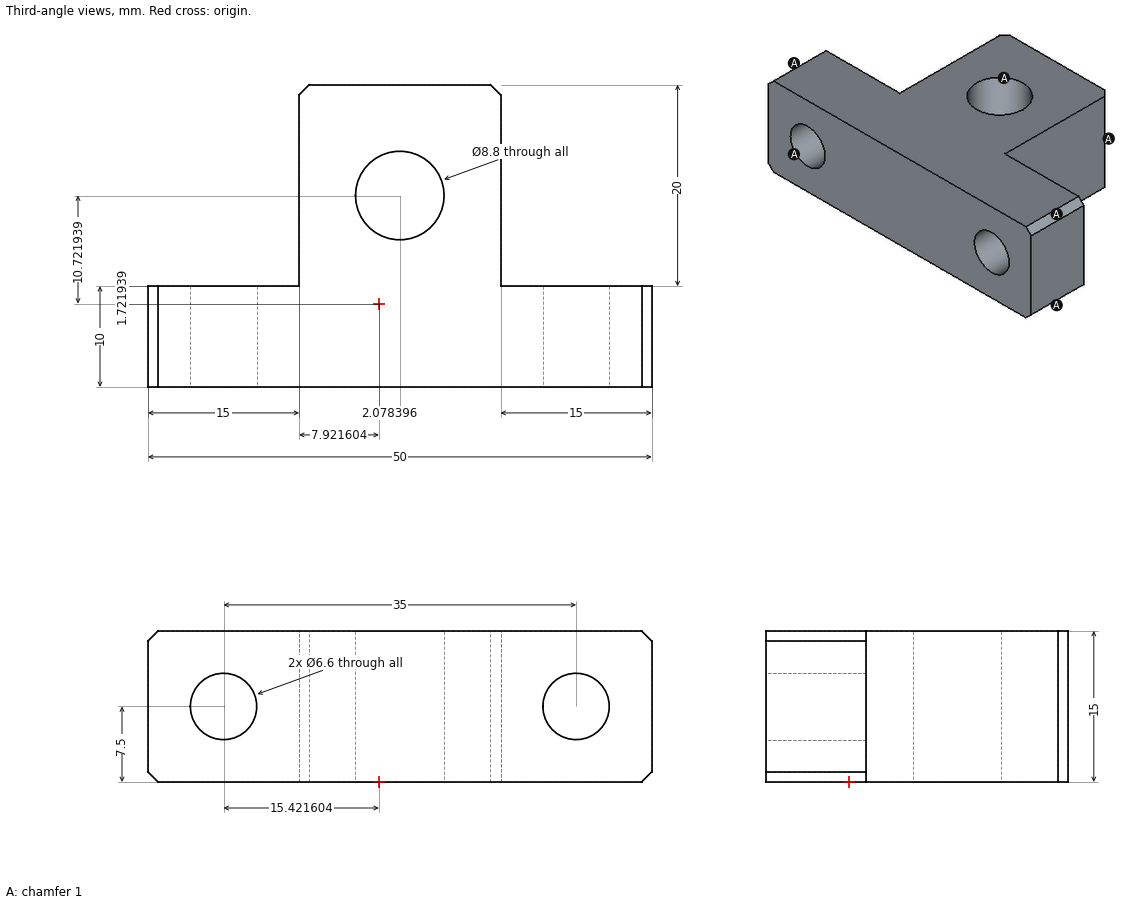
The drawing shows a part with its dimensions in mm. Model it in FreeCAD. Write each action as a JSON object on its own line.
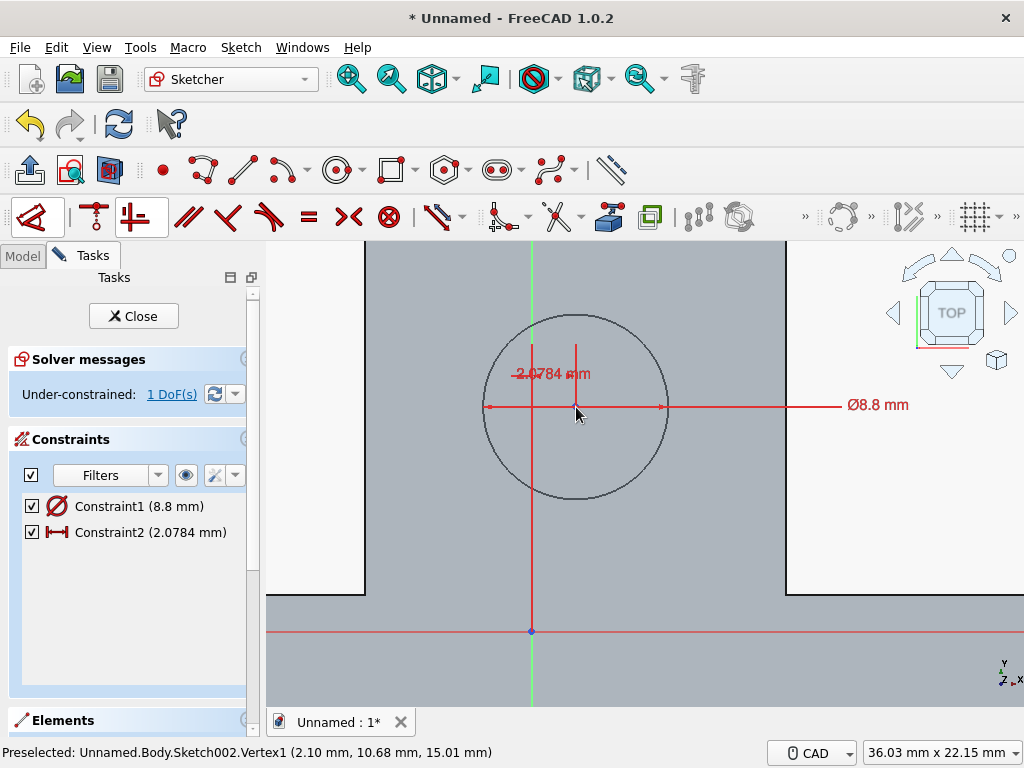
{"action": "left_click", "coordinate": [576, 407]}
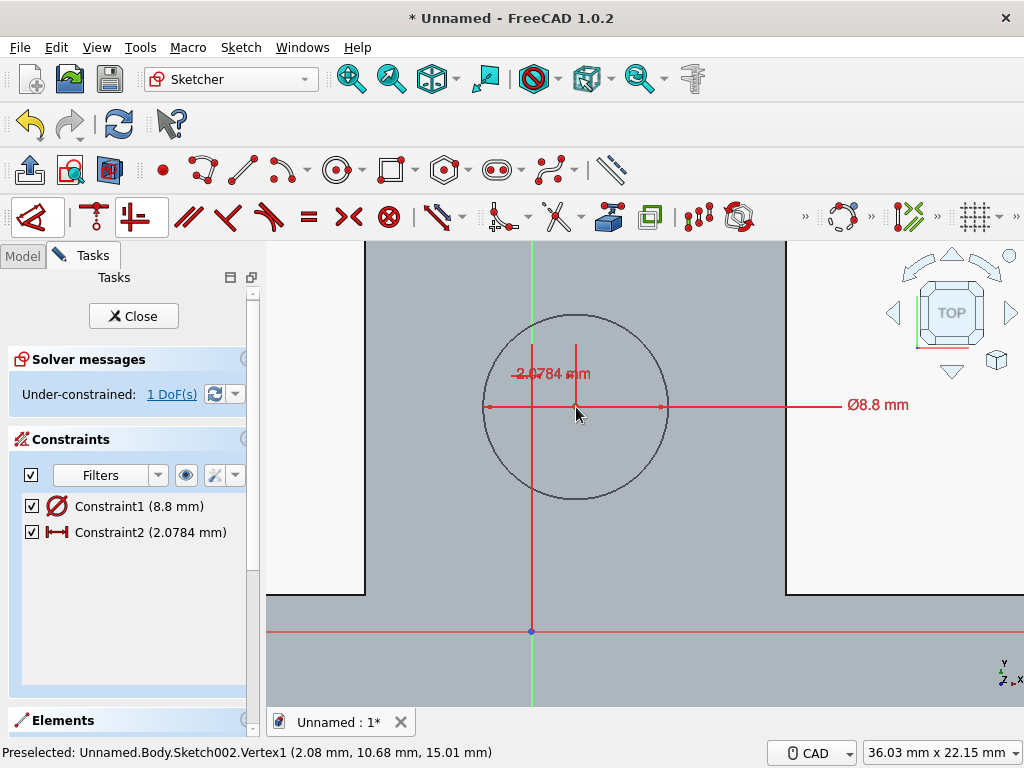
{"action": "left_click", "coordinate": [58, 218]}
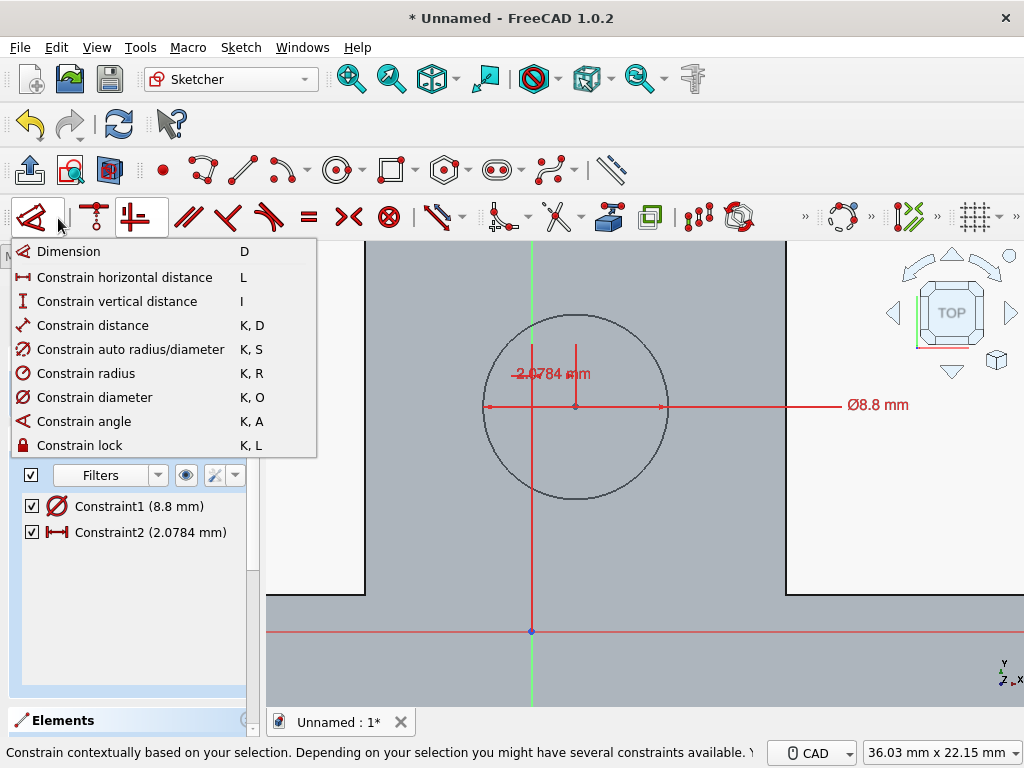
{"action": "left_click", "coordinate": [164, 301]}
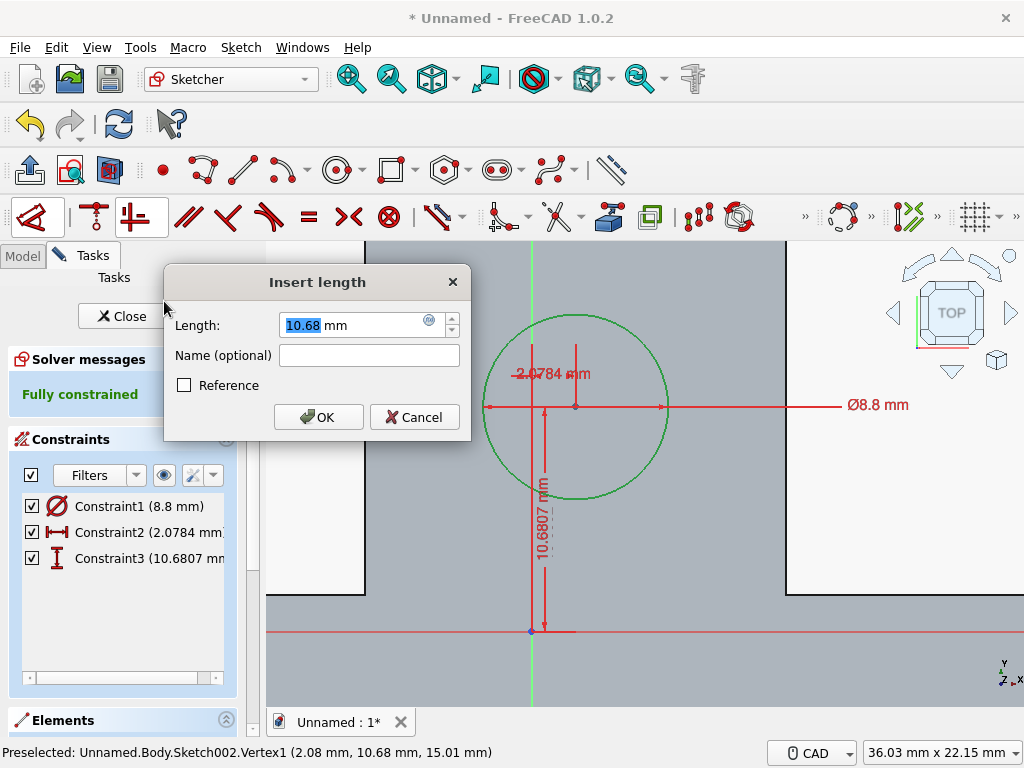
{"action": "type", "text": "10.721939"}
{"action": "key", "text": "Return"}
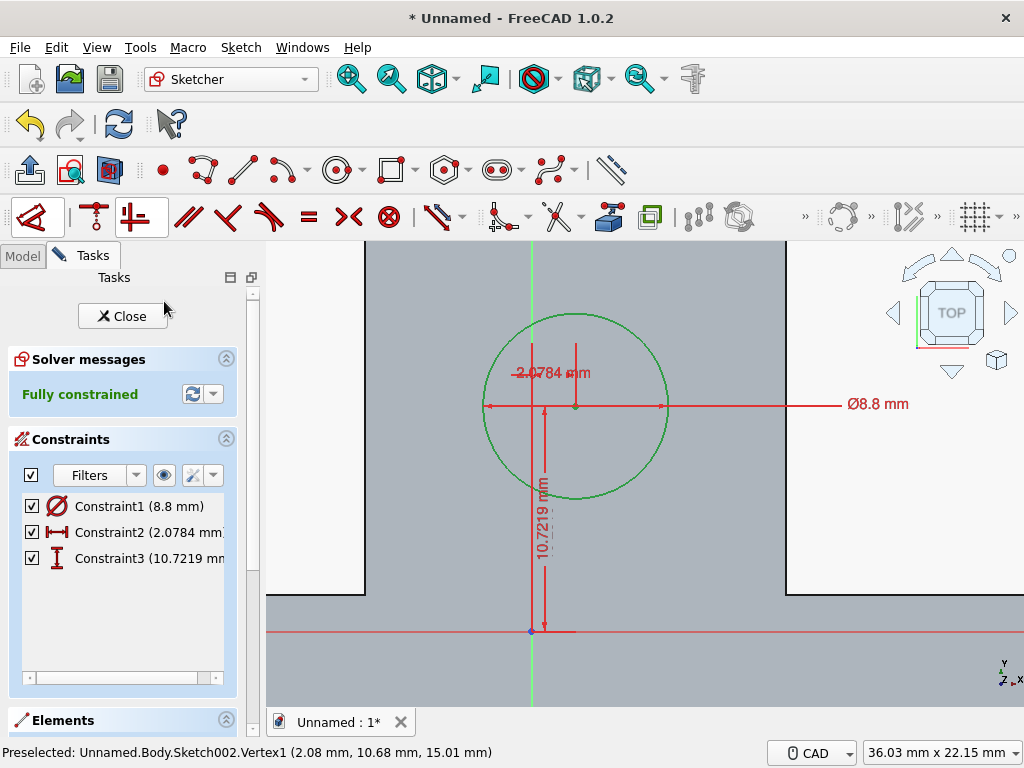
{"action": "left_click", "coordinate": [123, 316]}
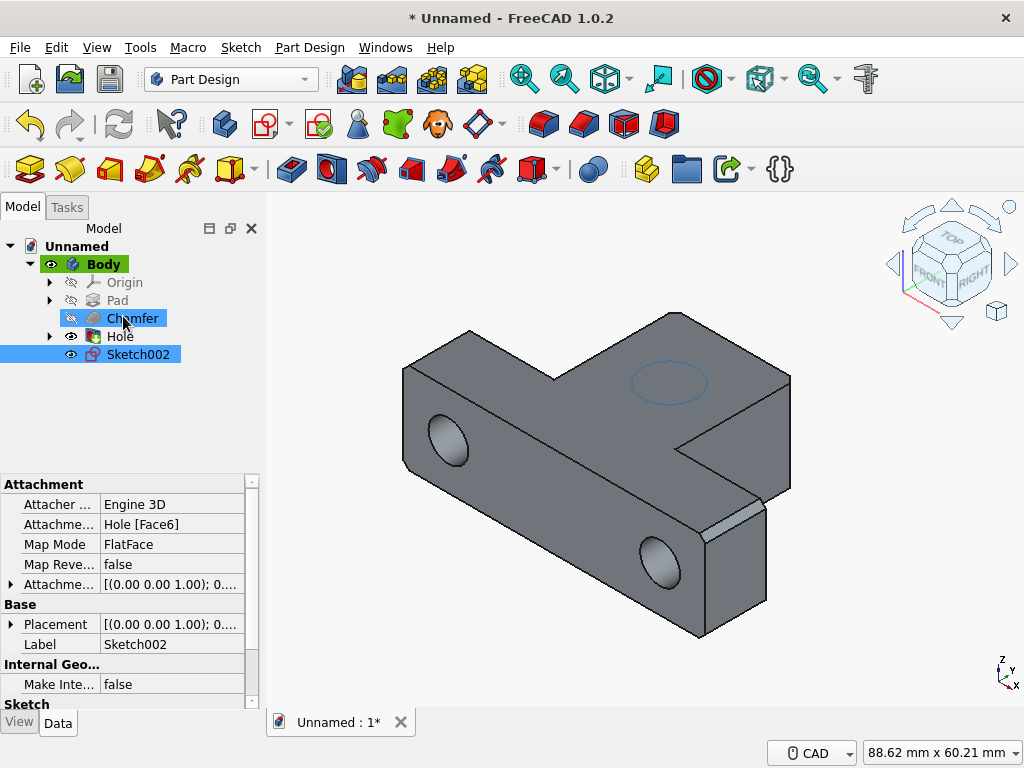
{"action": "left_click", "coordinate": [332, 170]}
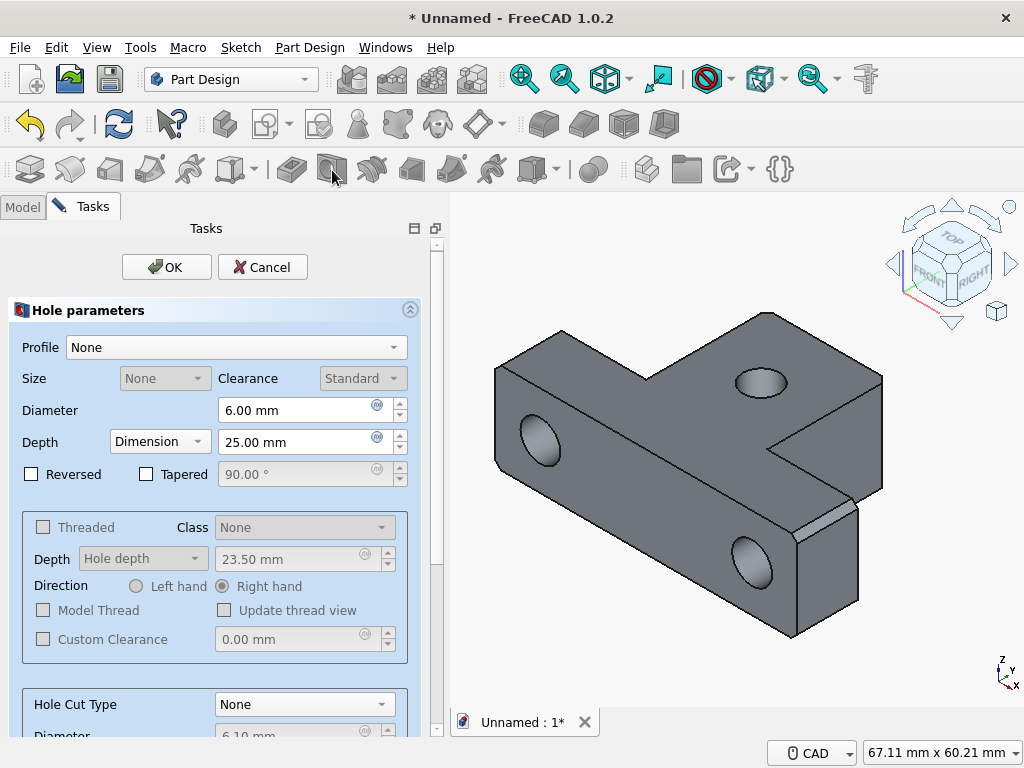
{"action": "triple_click", "coordinate": [305, 410]}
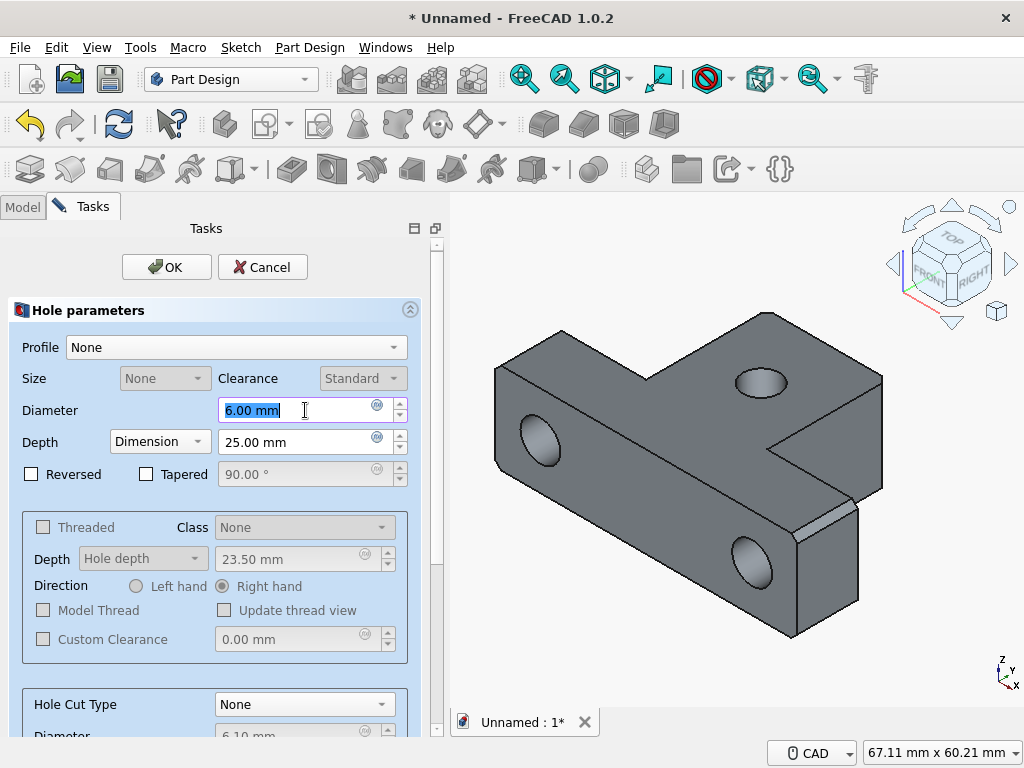
{"action": "type", "text": "8.8"}
{"action": "key", "text": "Tab"}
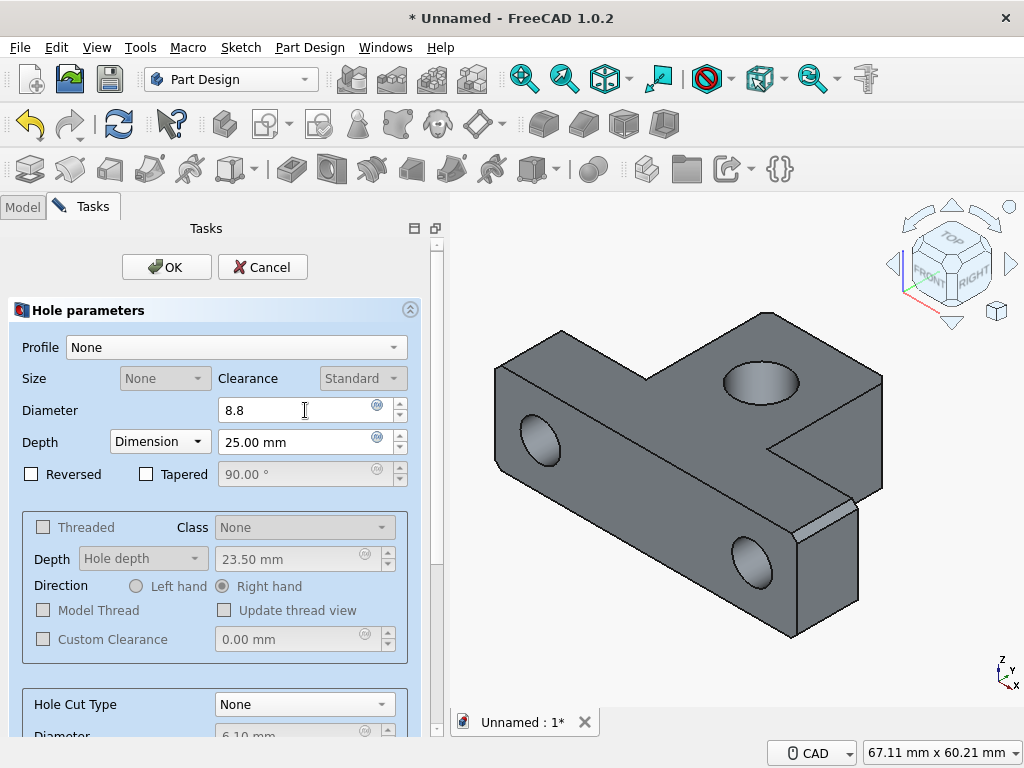
{"action": "left_click", "coordinate": [161, 442]}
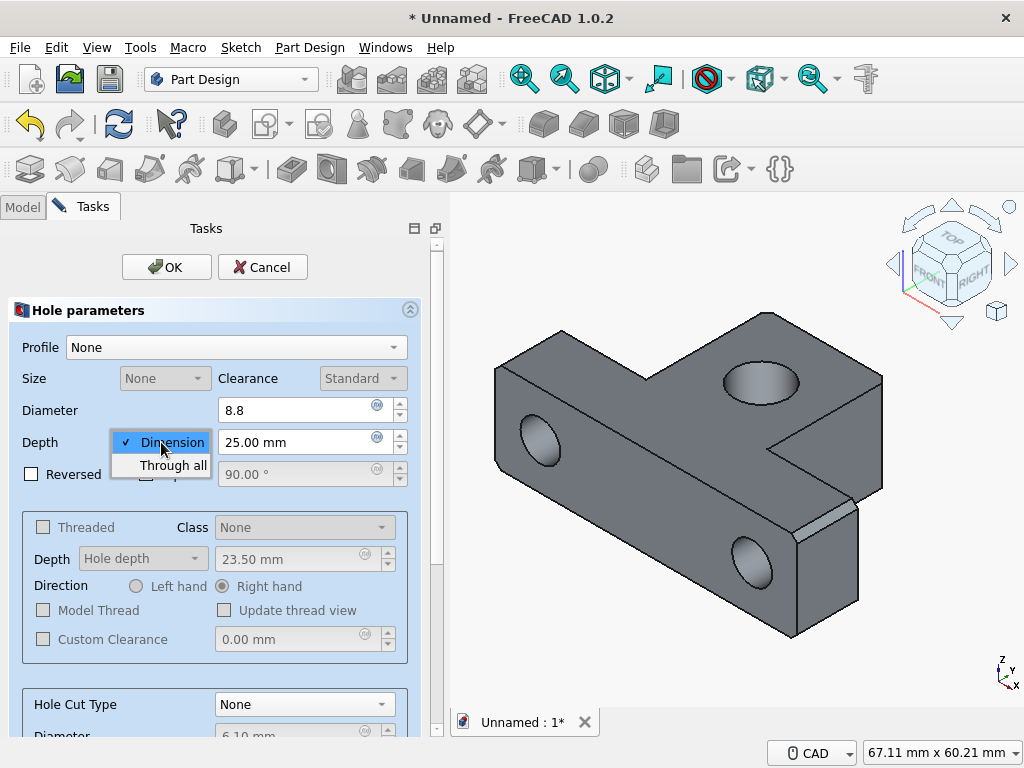
{"action": "left_click", "coordinate": [160, 466]}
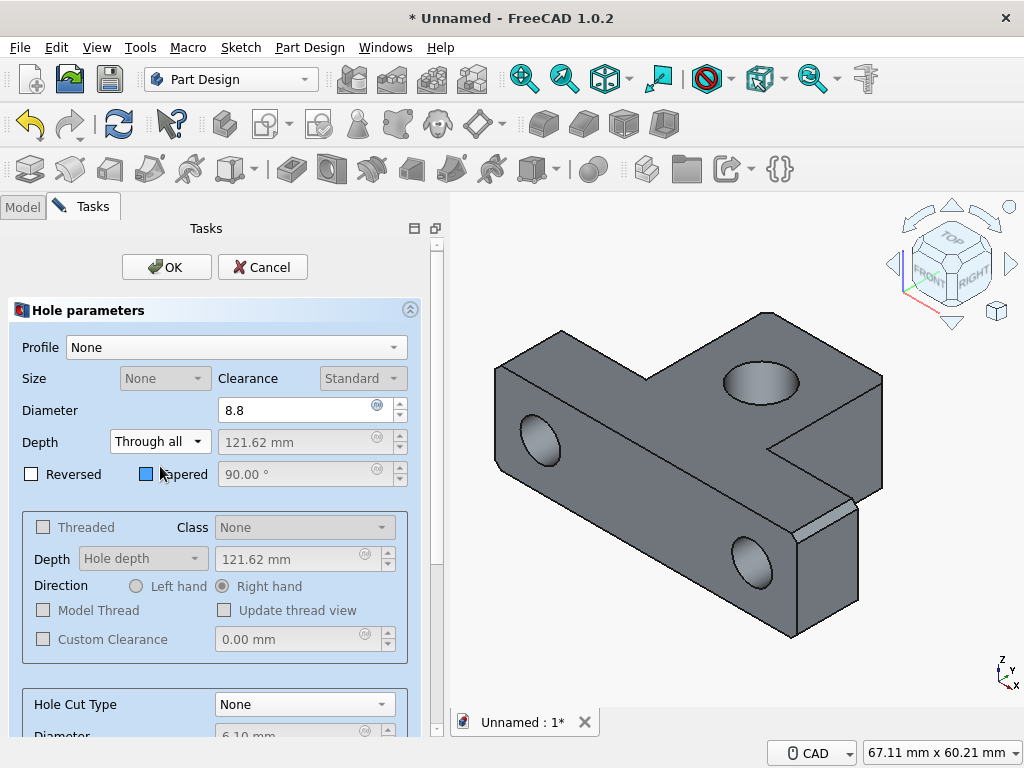
{"action": "left_click", "coordinate": [167, 267]}